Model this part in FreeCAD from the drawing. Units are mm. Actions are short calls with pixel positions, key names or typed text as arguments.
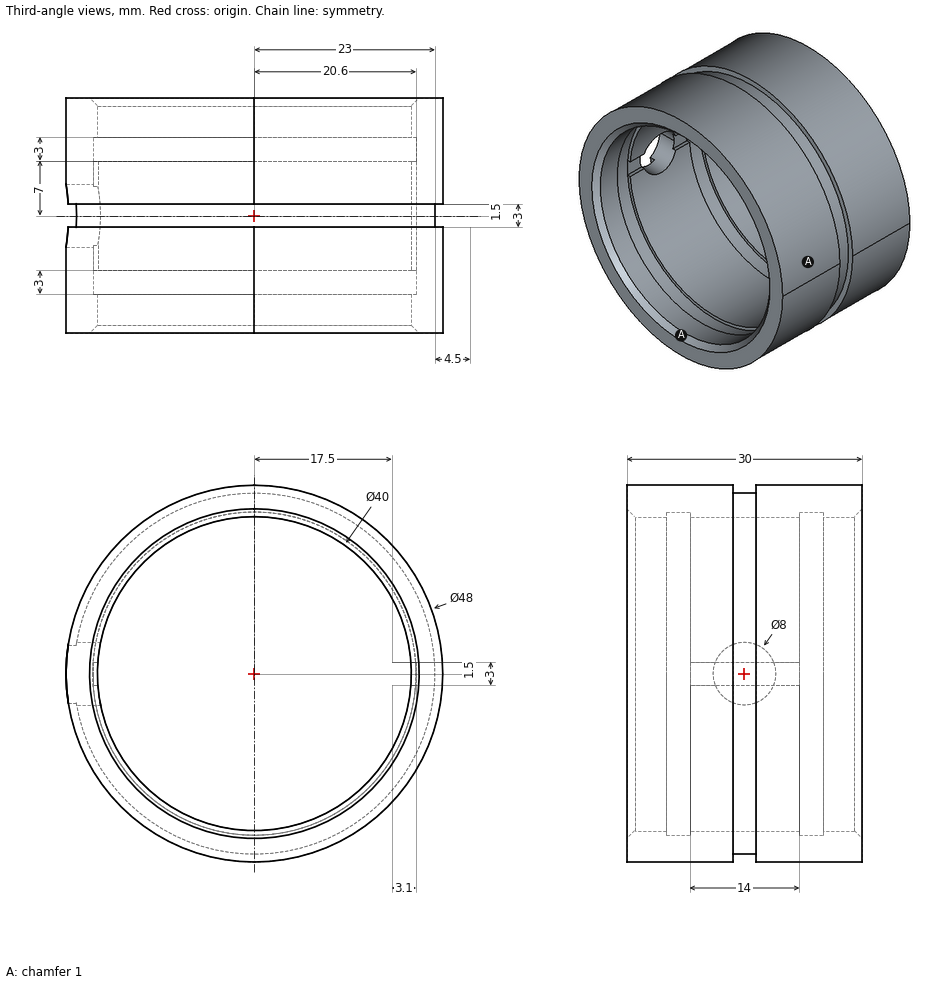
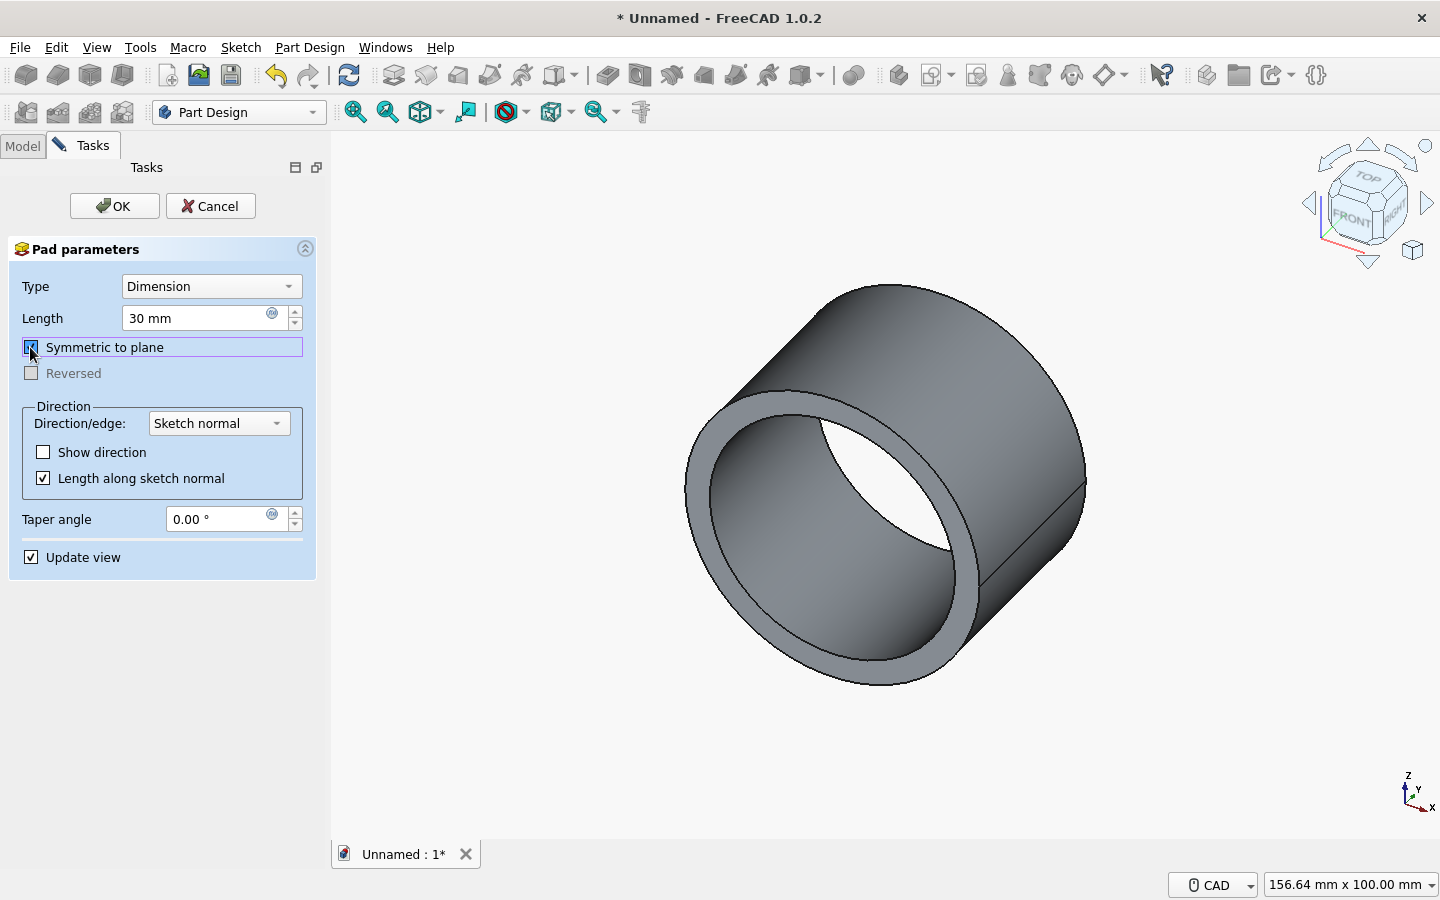
click(115, 206)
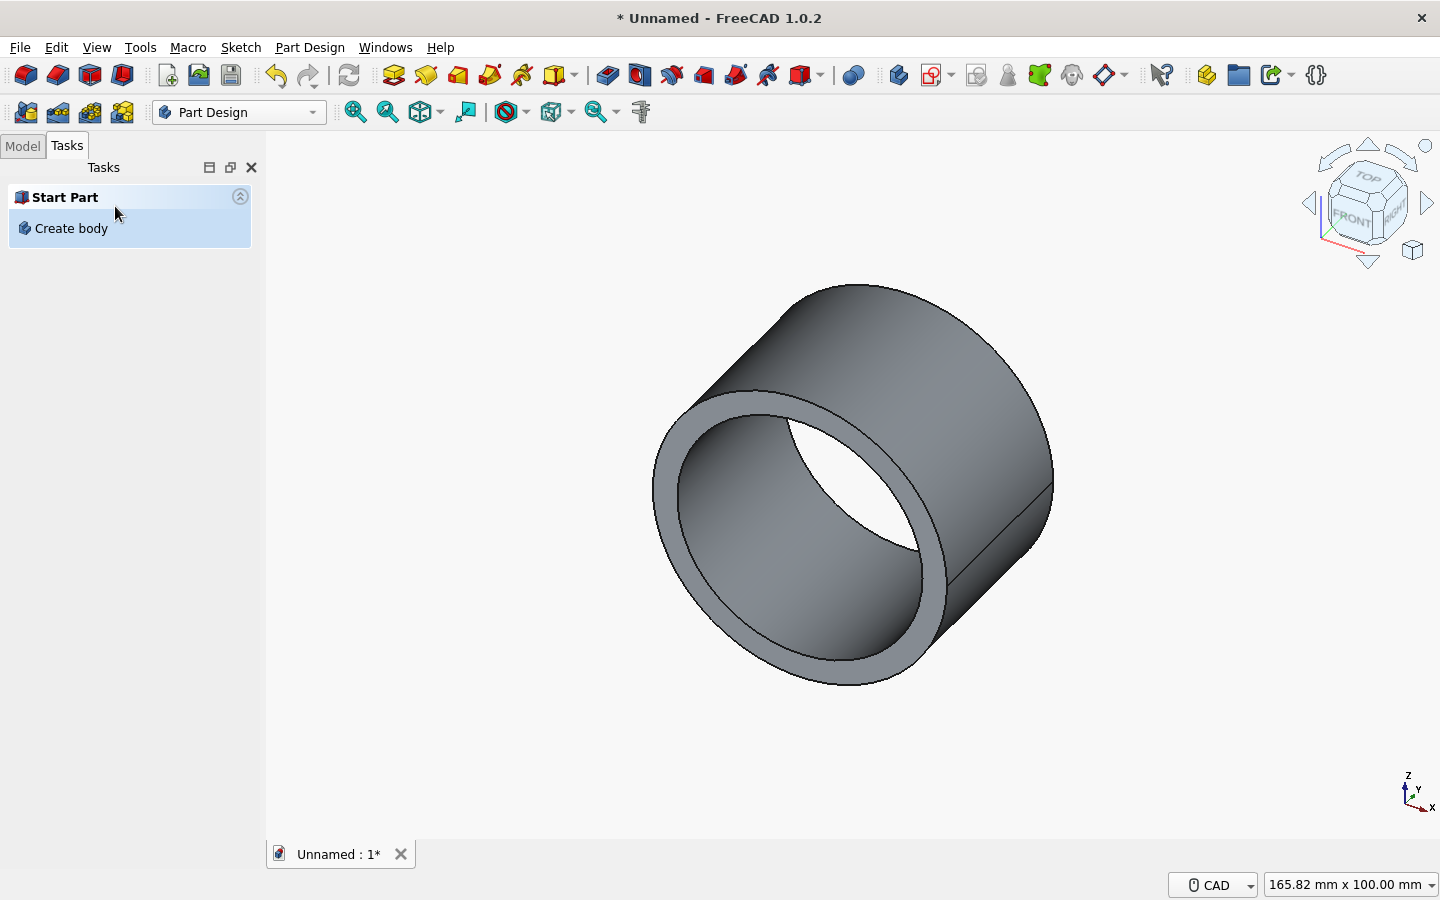
click(932, 76)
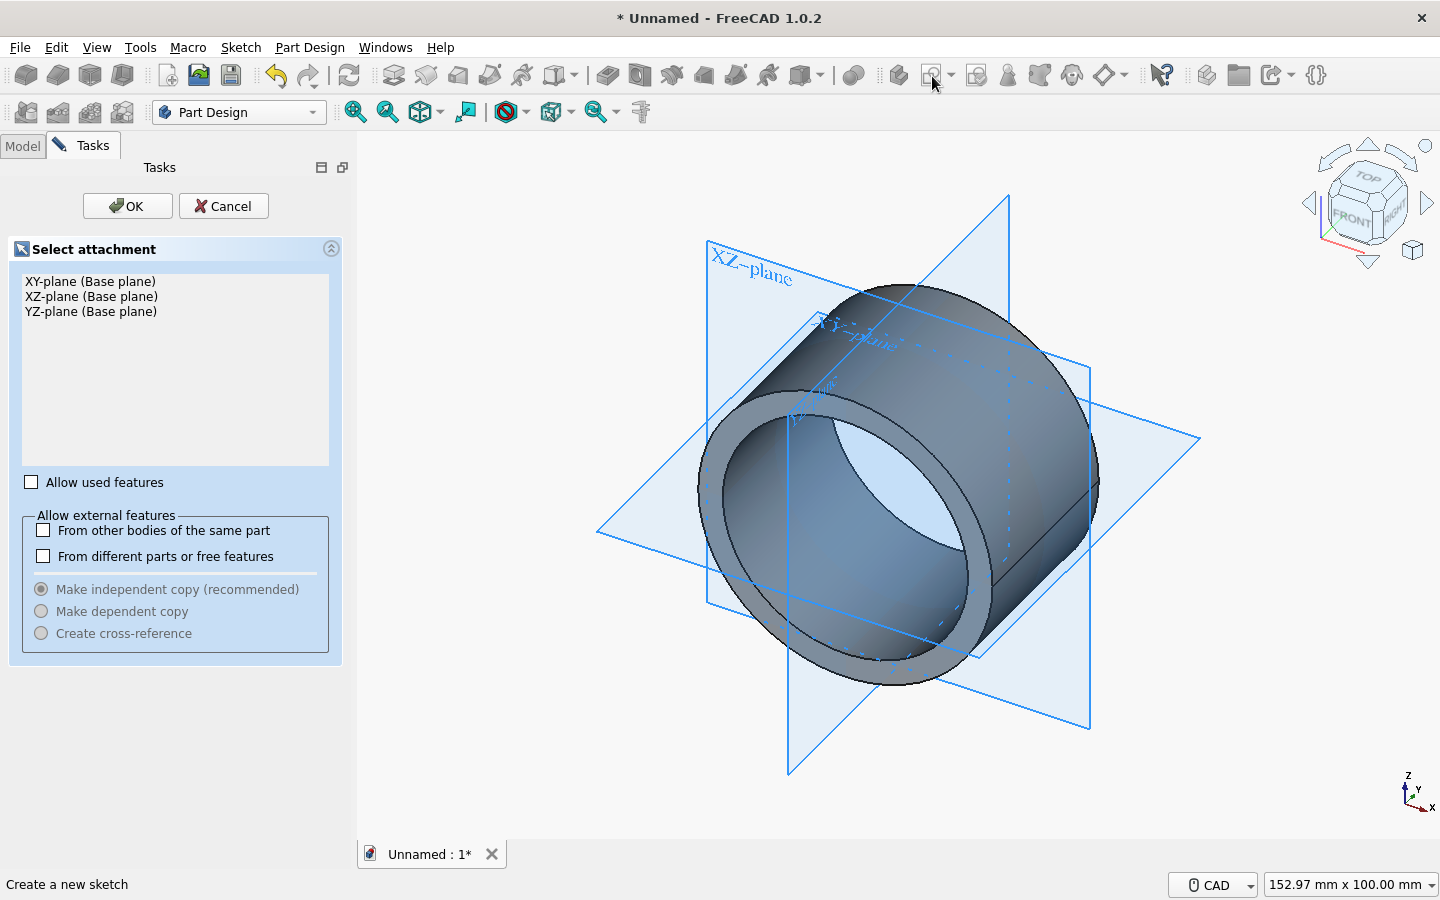
click(82, 282)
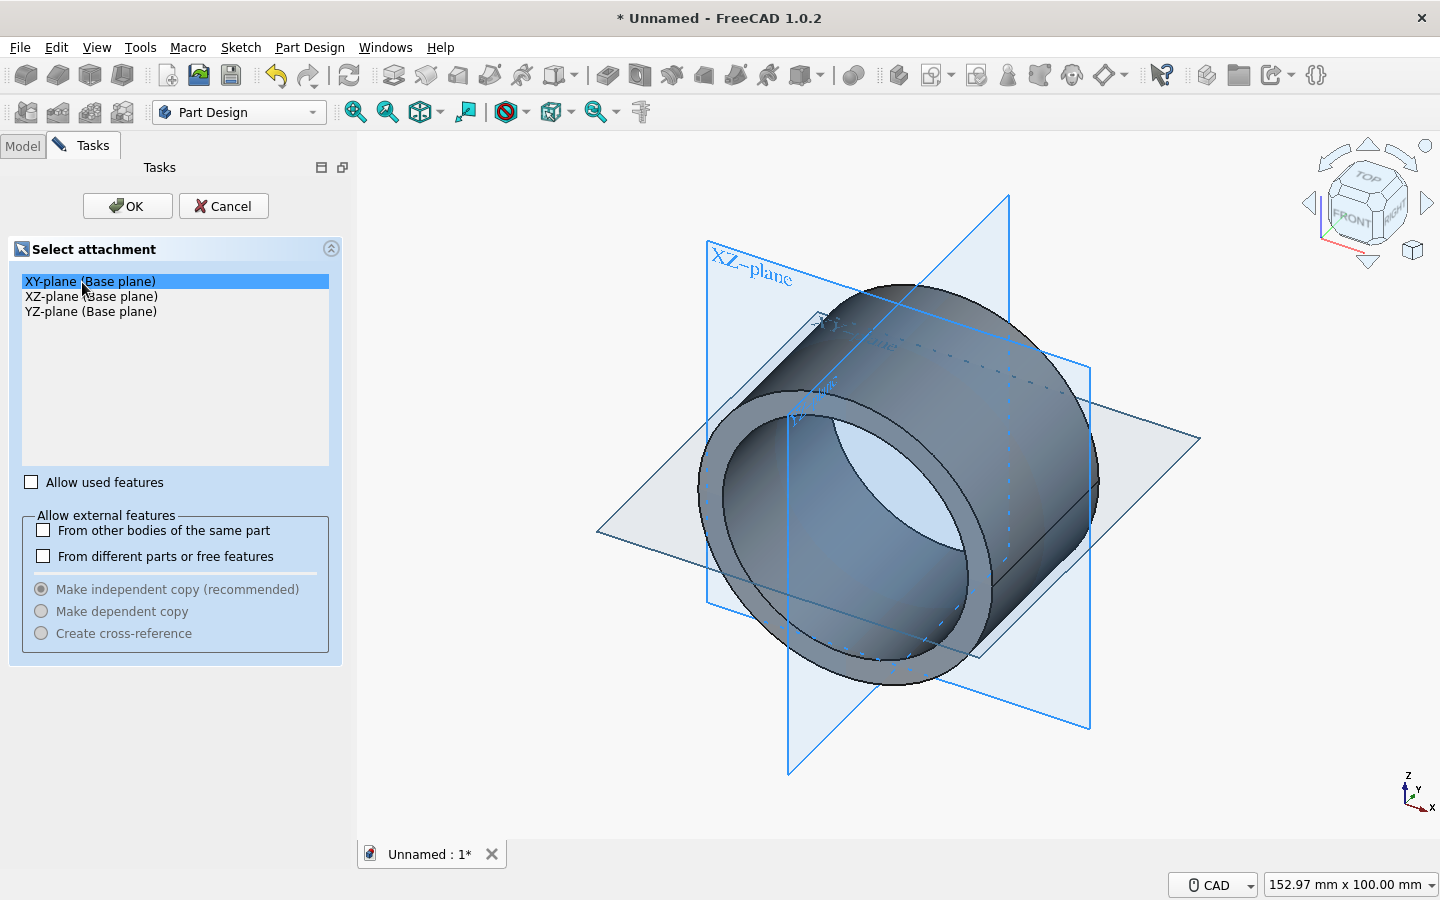
click(128, 206)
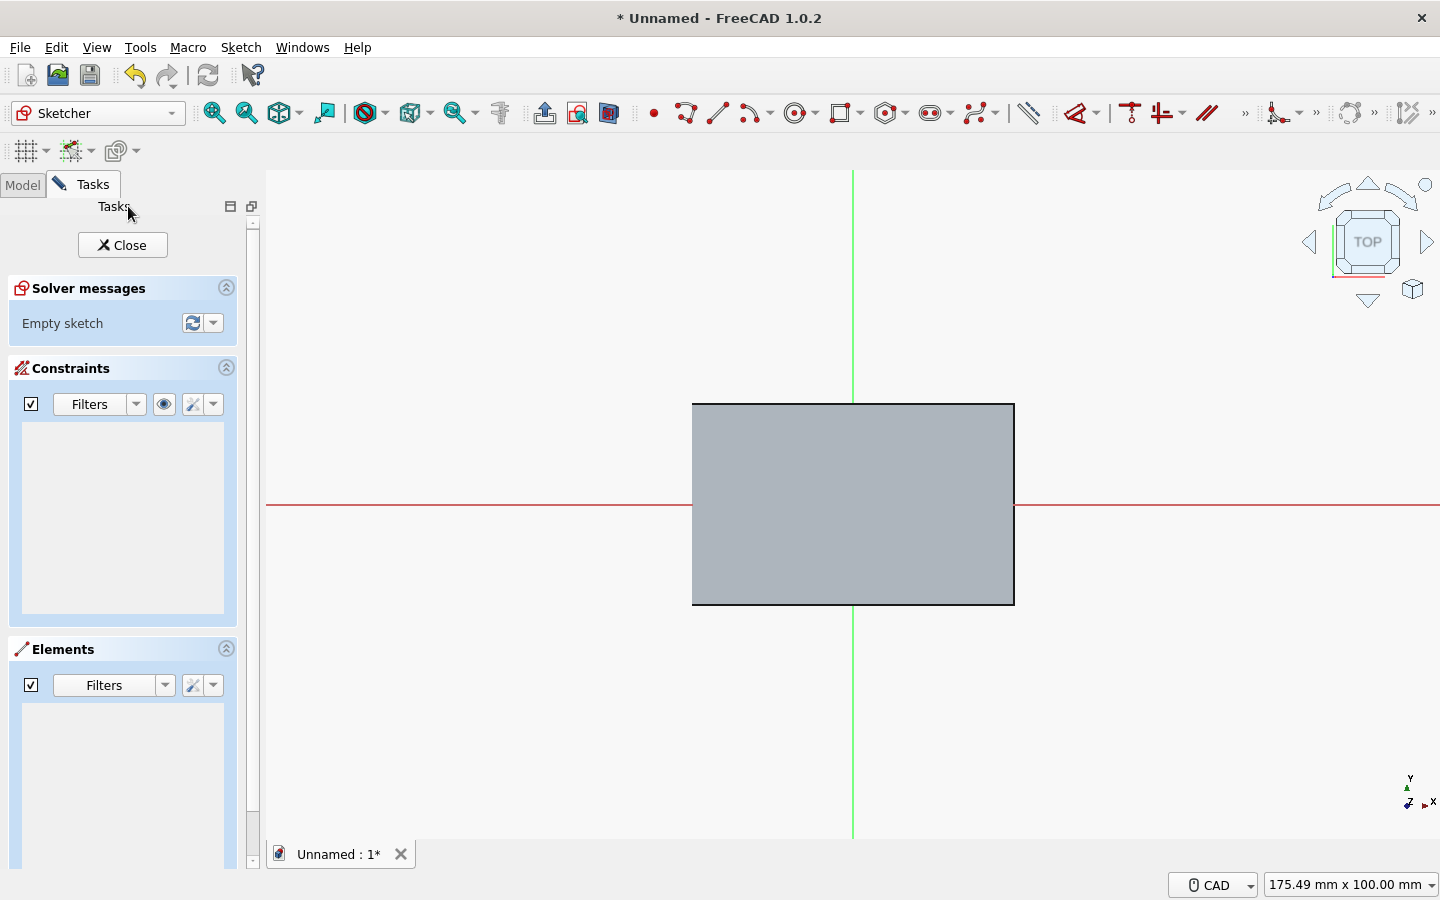
click(610, 114)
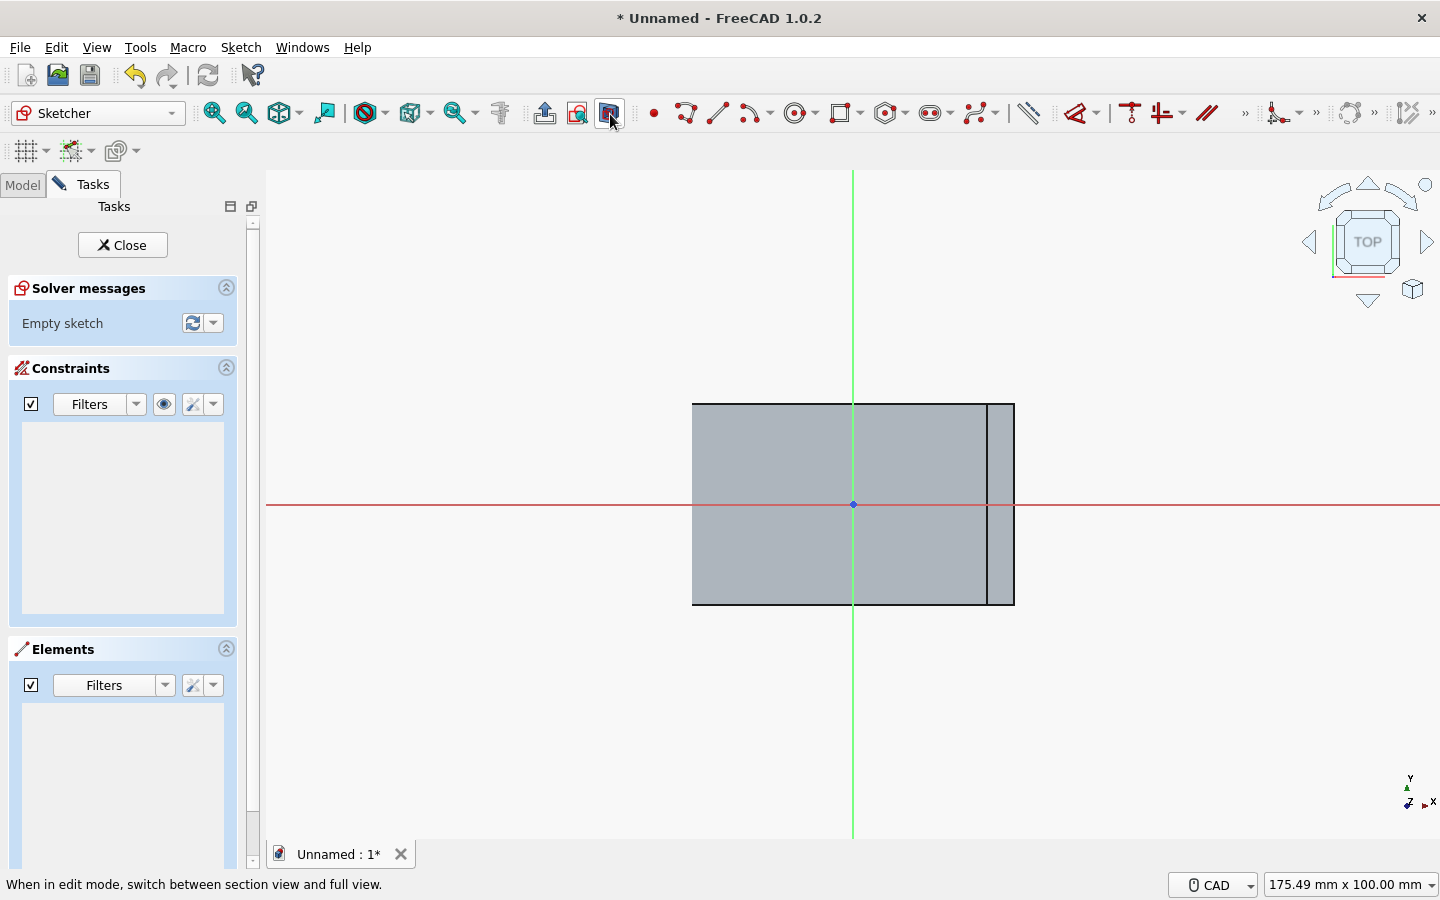
scroll(1014, 504, up, 6)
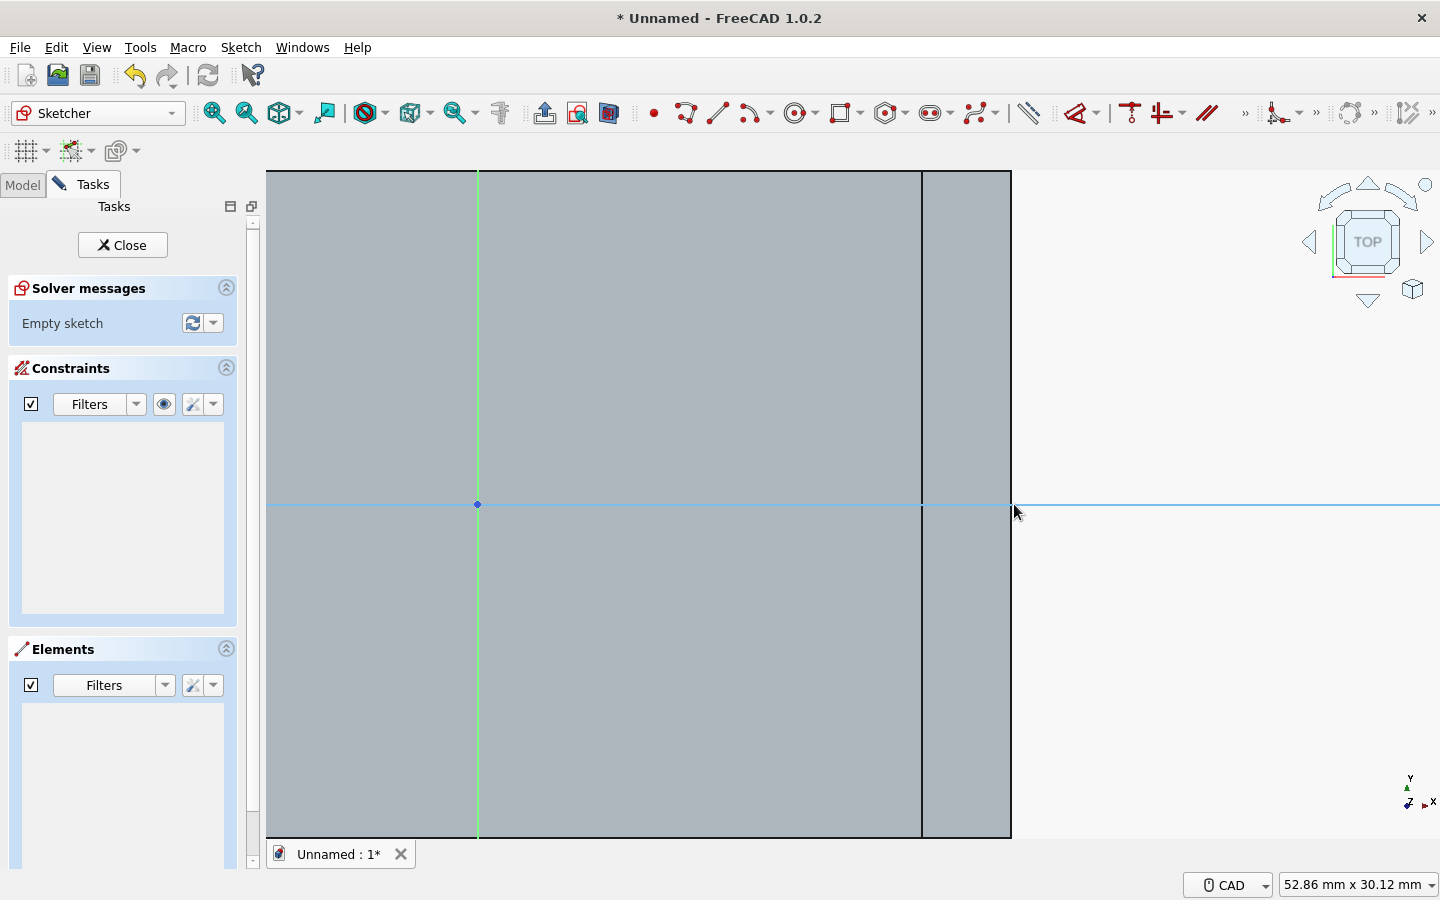
click(840, 114)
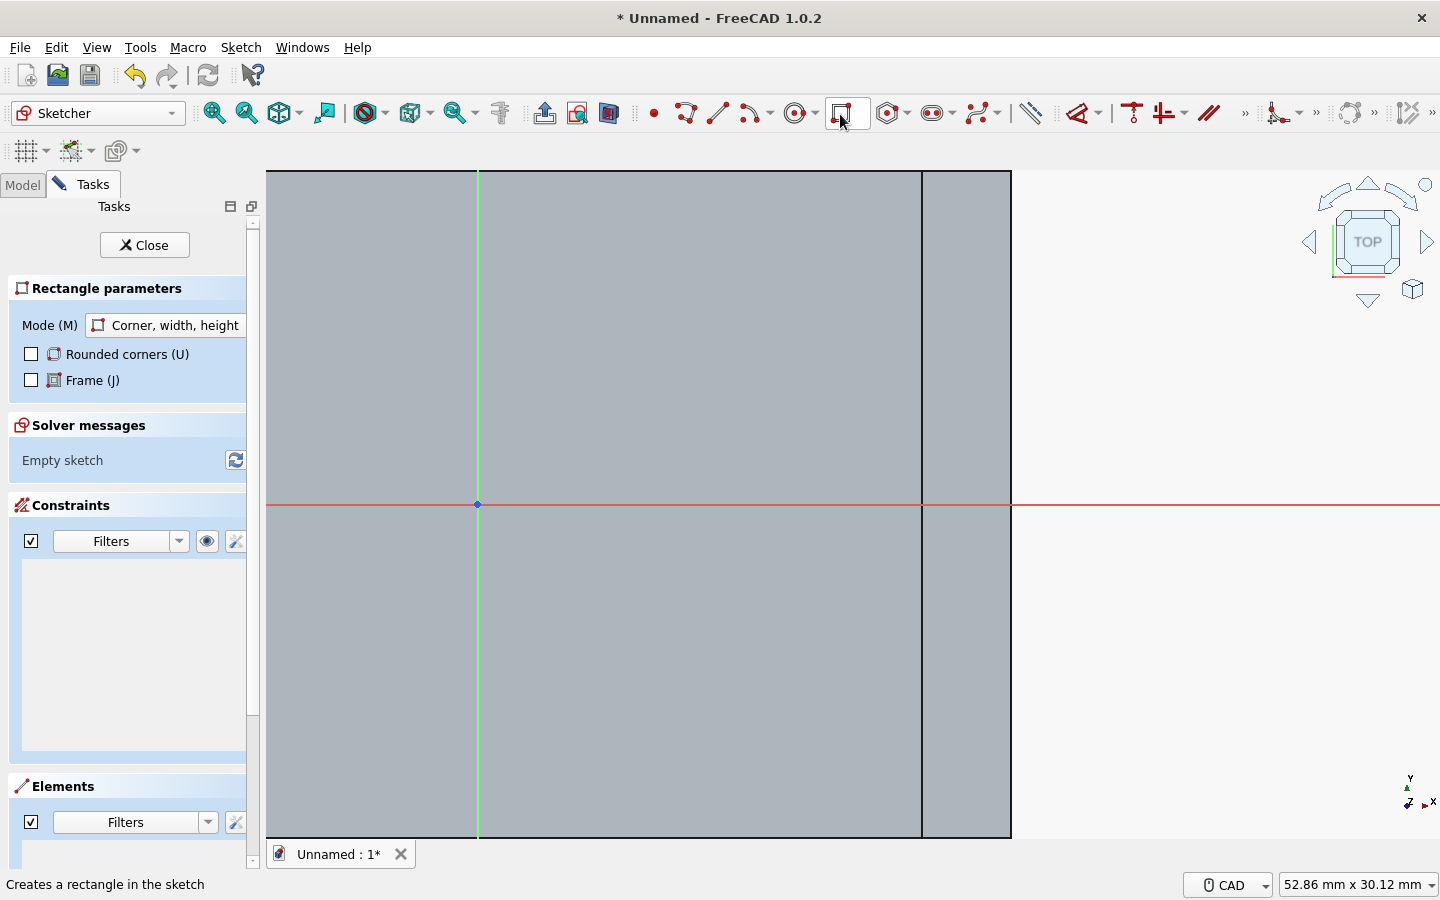
click(478, 282)
click(936, 349)